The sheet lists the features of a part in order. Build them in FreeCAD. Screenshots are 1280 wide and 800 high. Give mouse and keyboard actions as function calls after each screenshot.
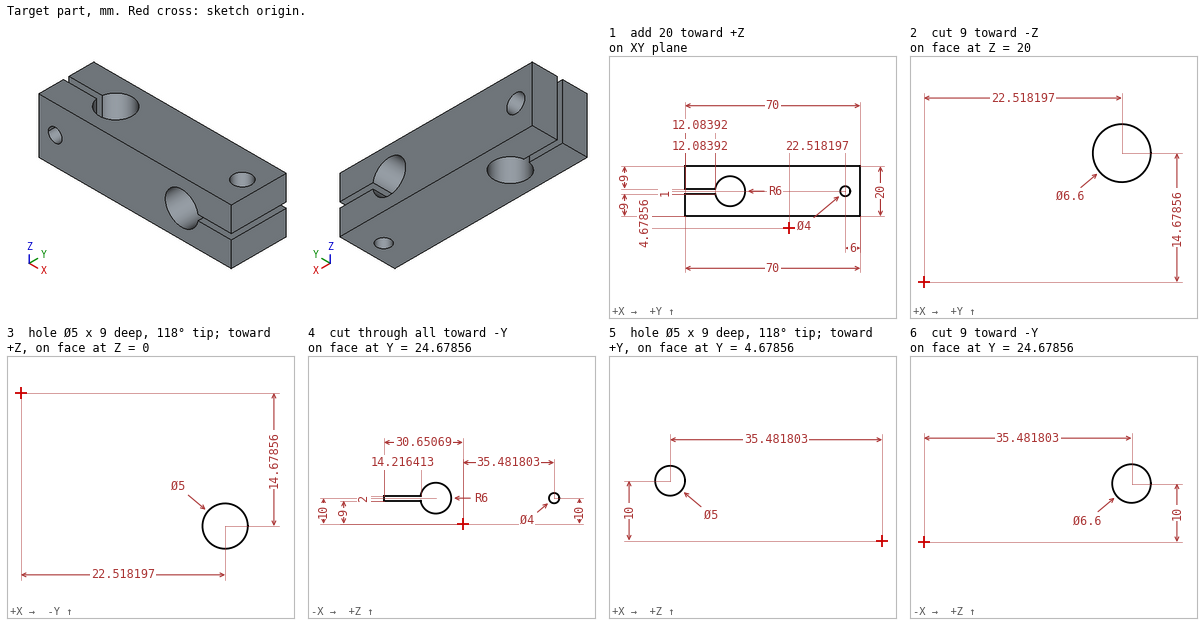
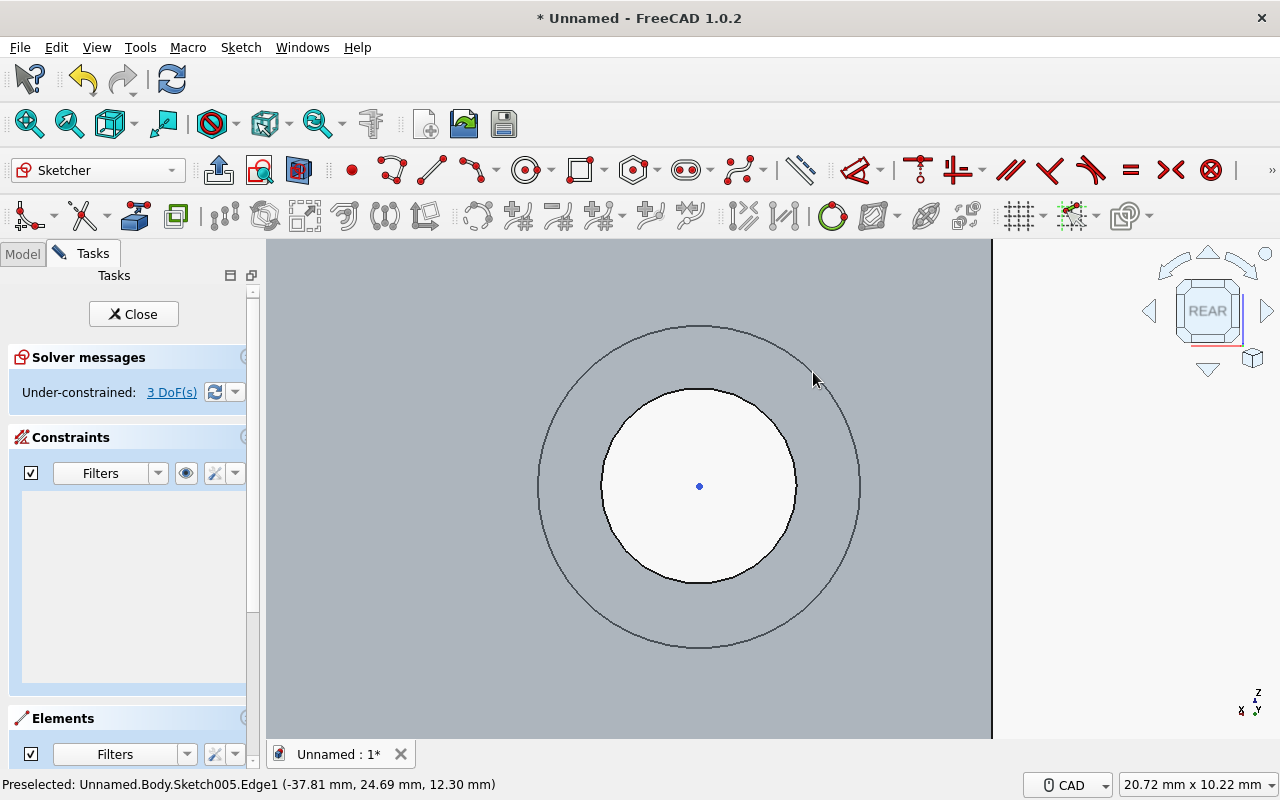
click(856, 170)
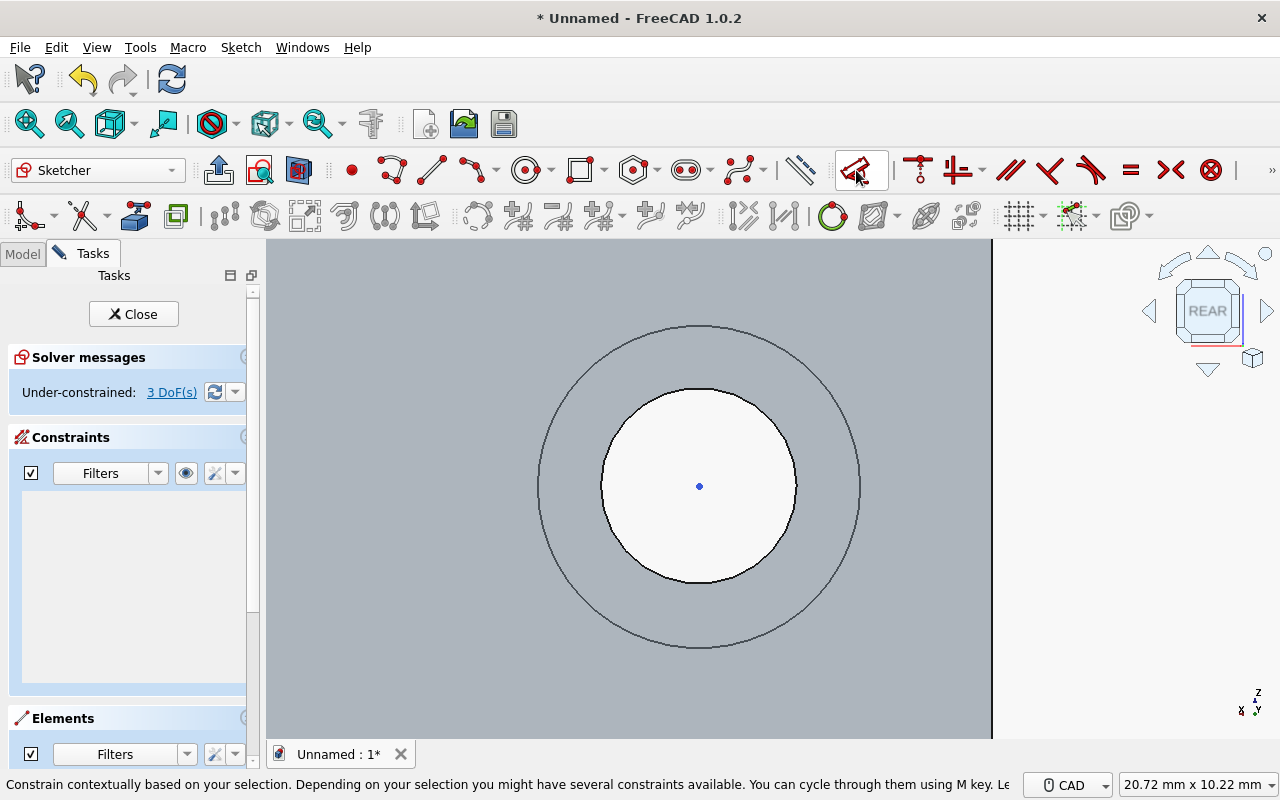
click(813, 373)
click(836, 350)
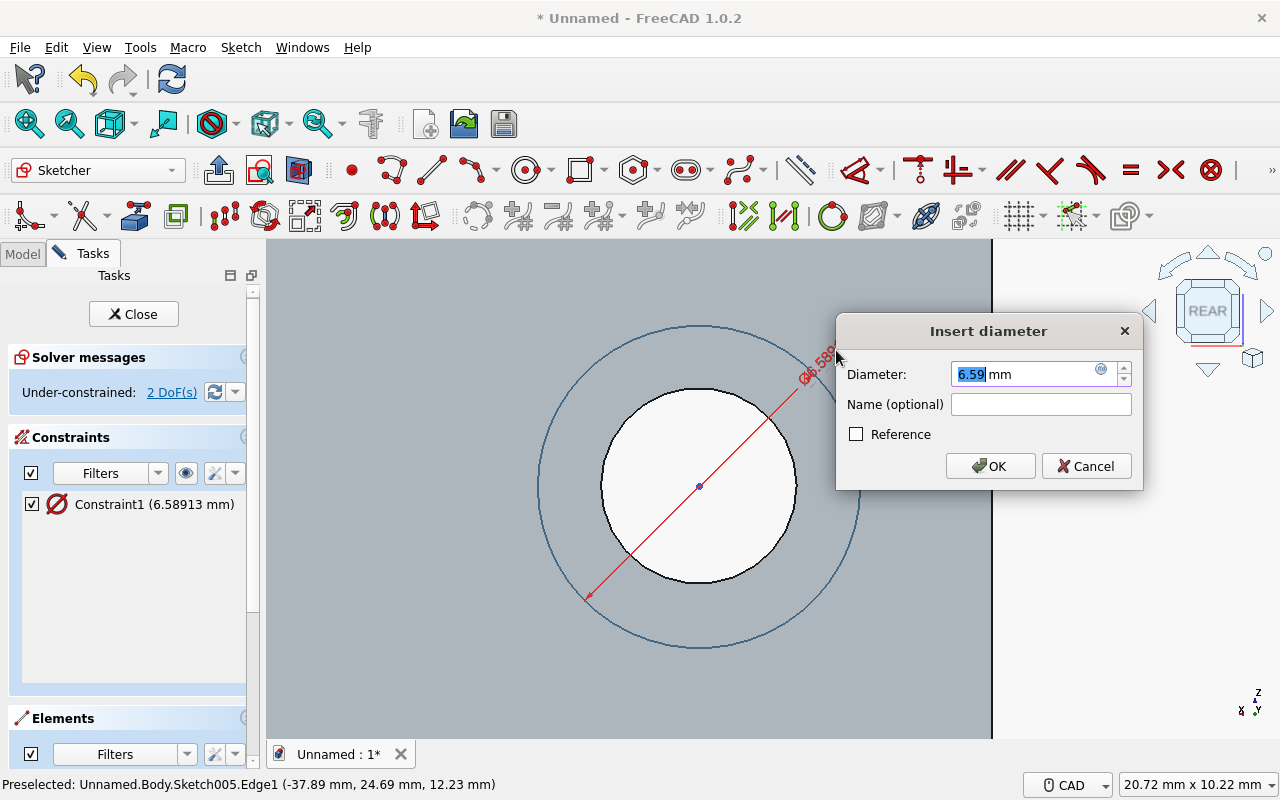
text(6.6)
key(Return)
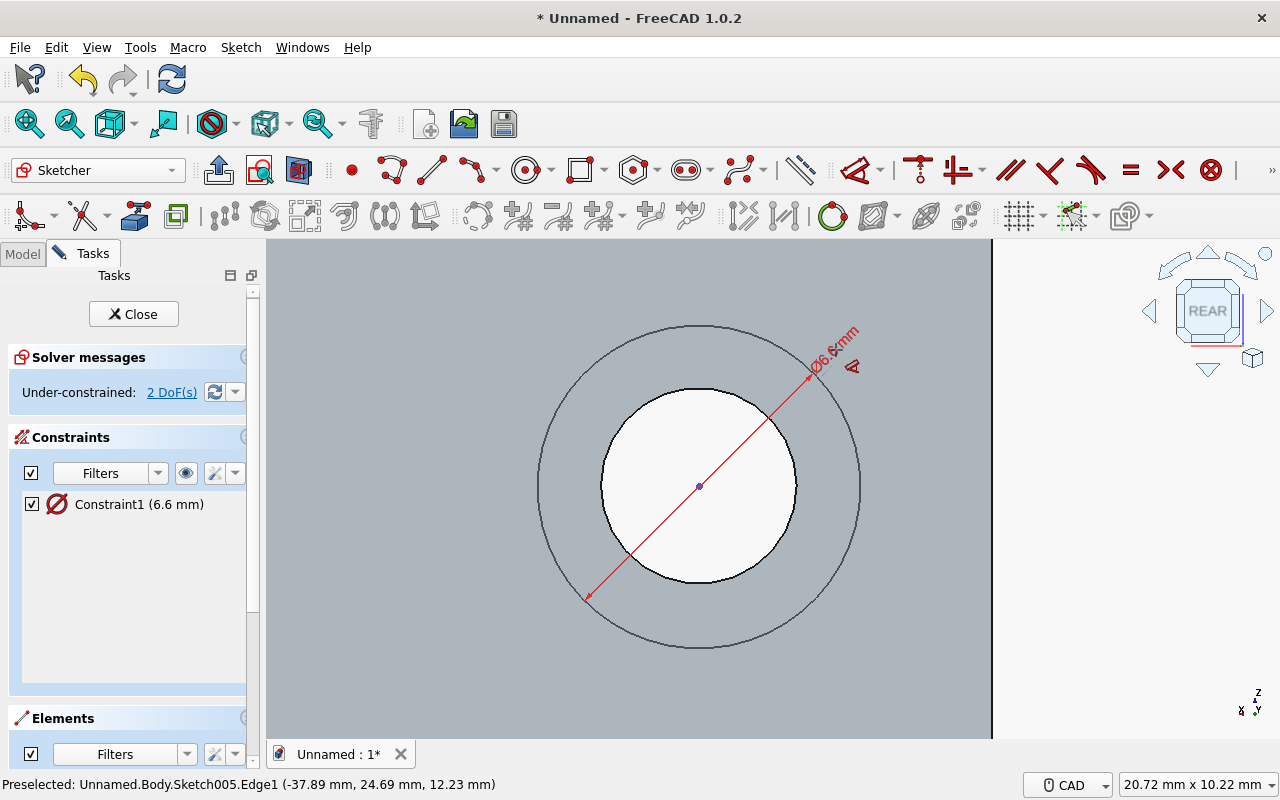
click(699, 487)
click(733, 599)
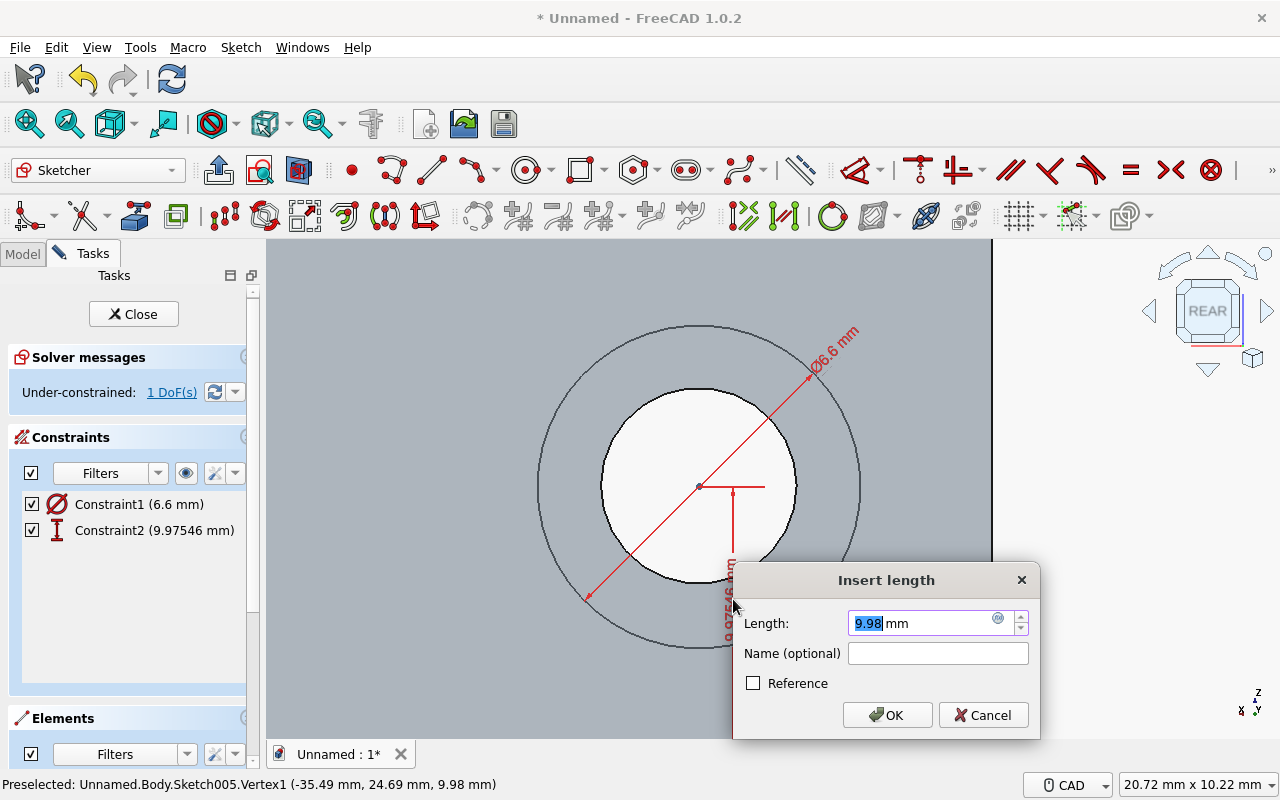
text(10)
key(Return)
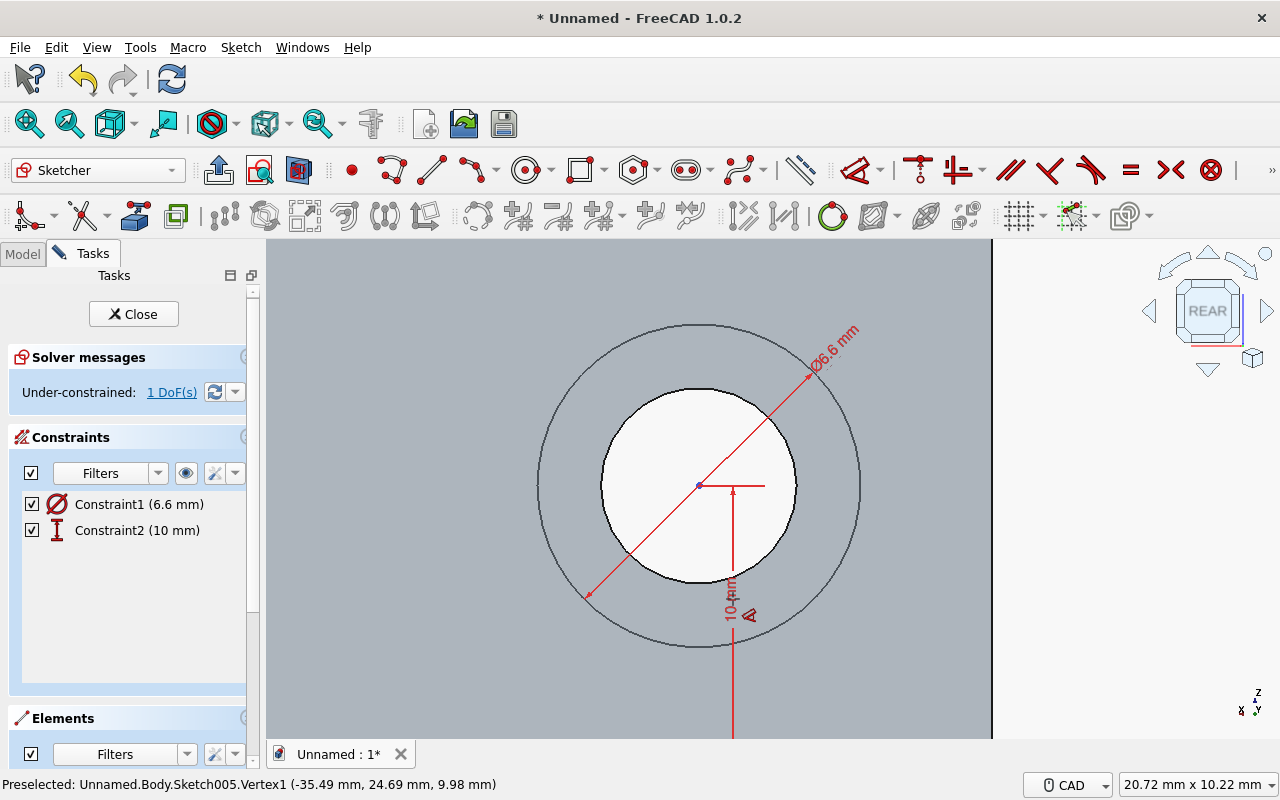
click(699, 486)
click(497, 452)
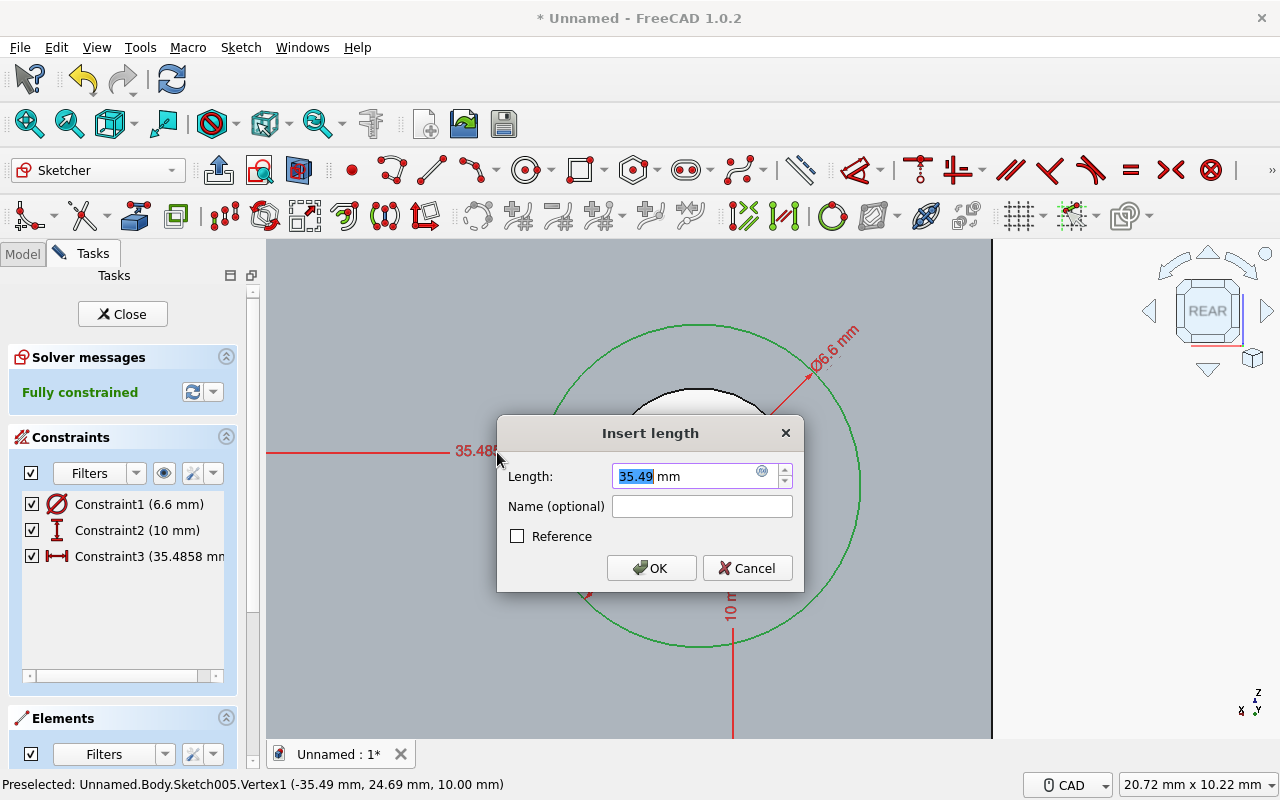
text(35.481803)
key(Return)
key(Escape)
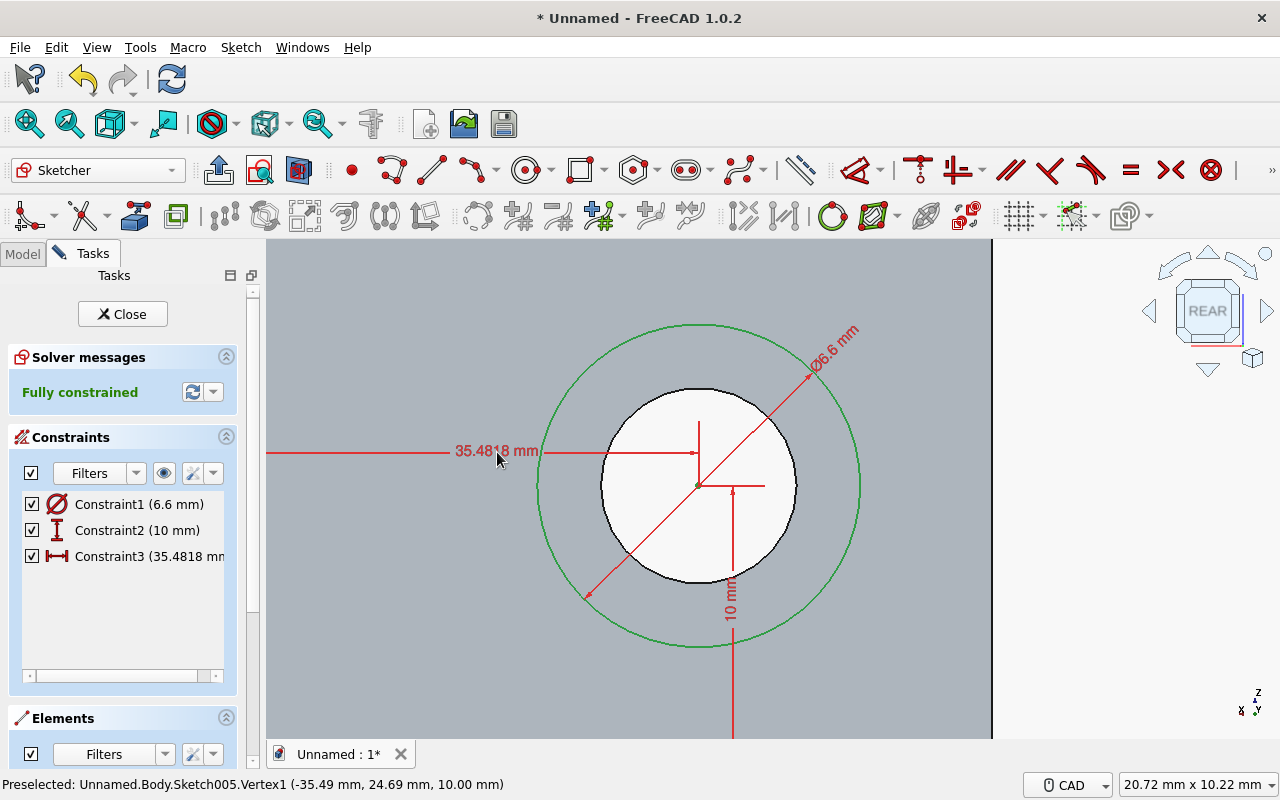
click(123, 314)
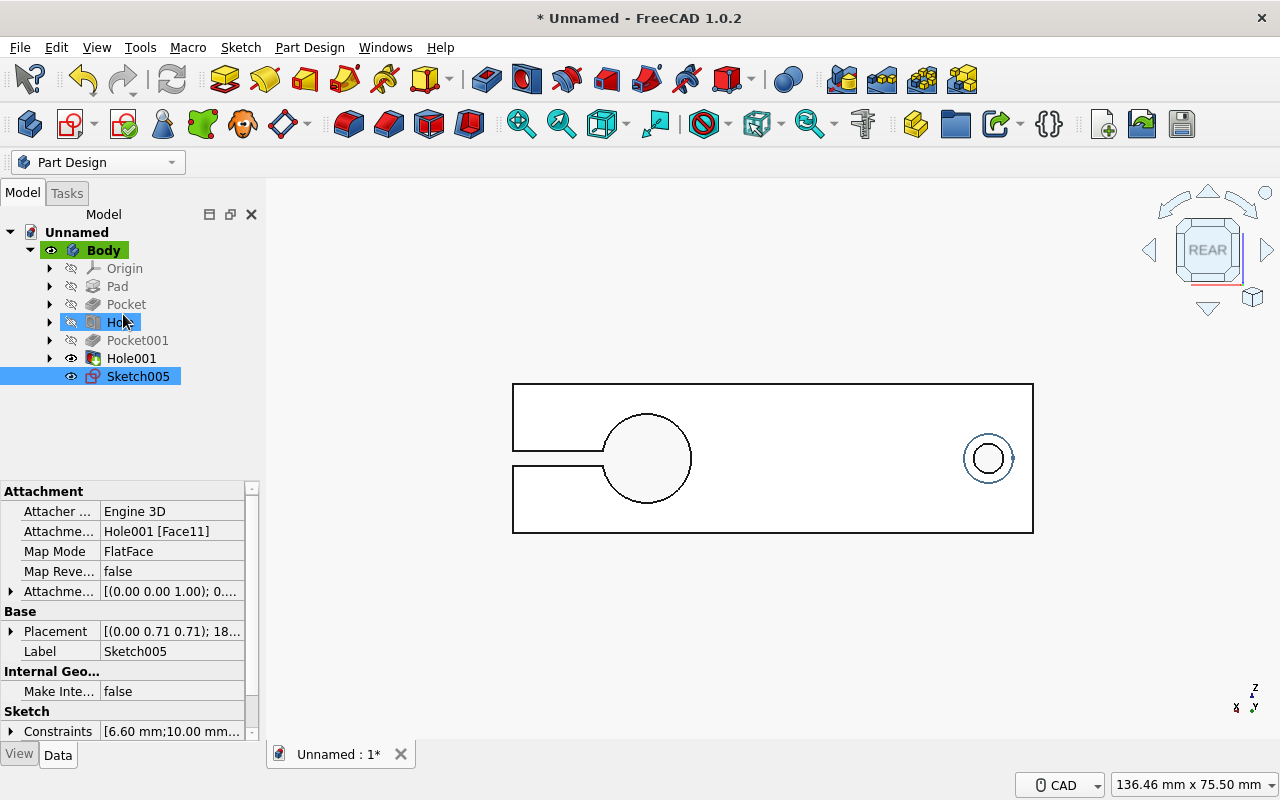
click(488, 80)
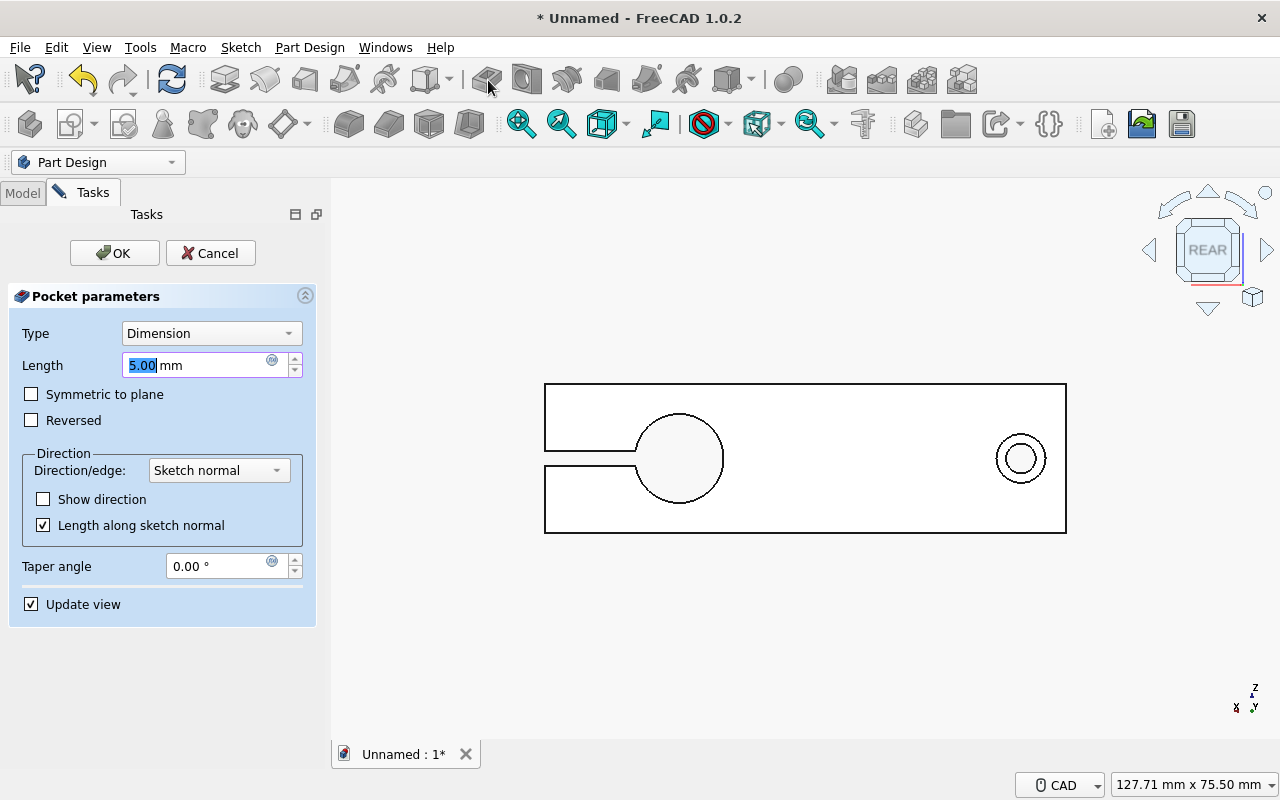
text(9)
key(Tab)